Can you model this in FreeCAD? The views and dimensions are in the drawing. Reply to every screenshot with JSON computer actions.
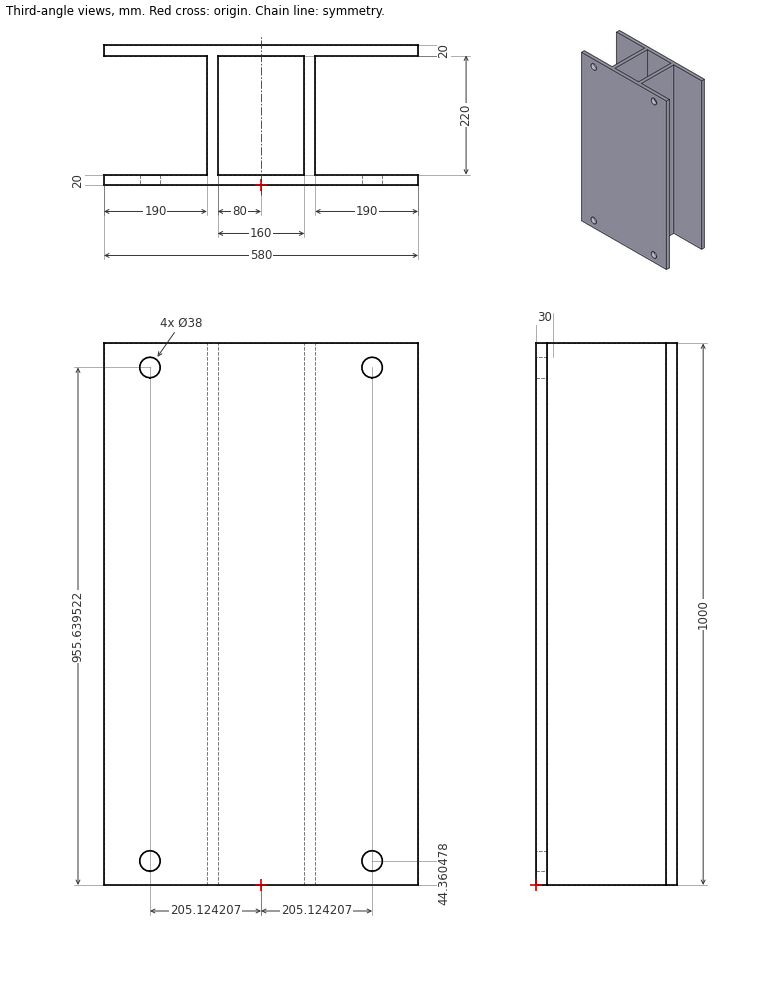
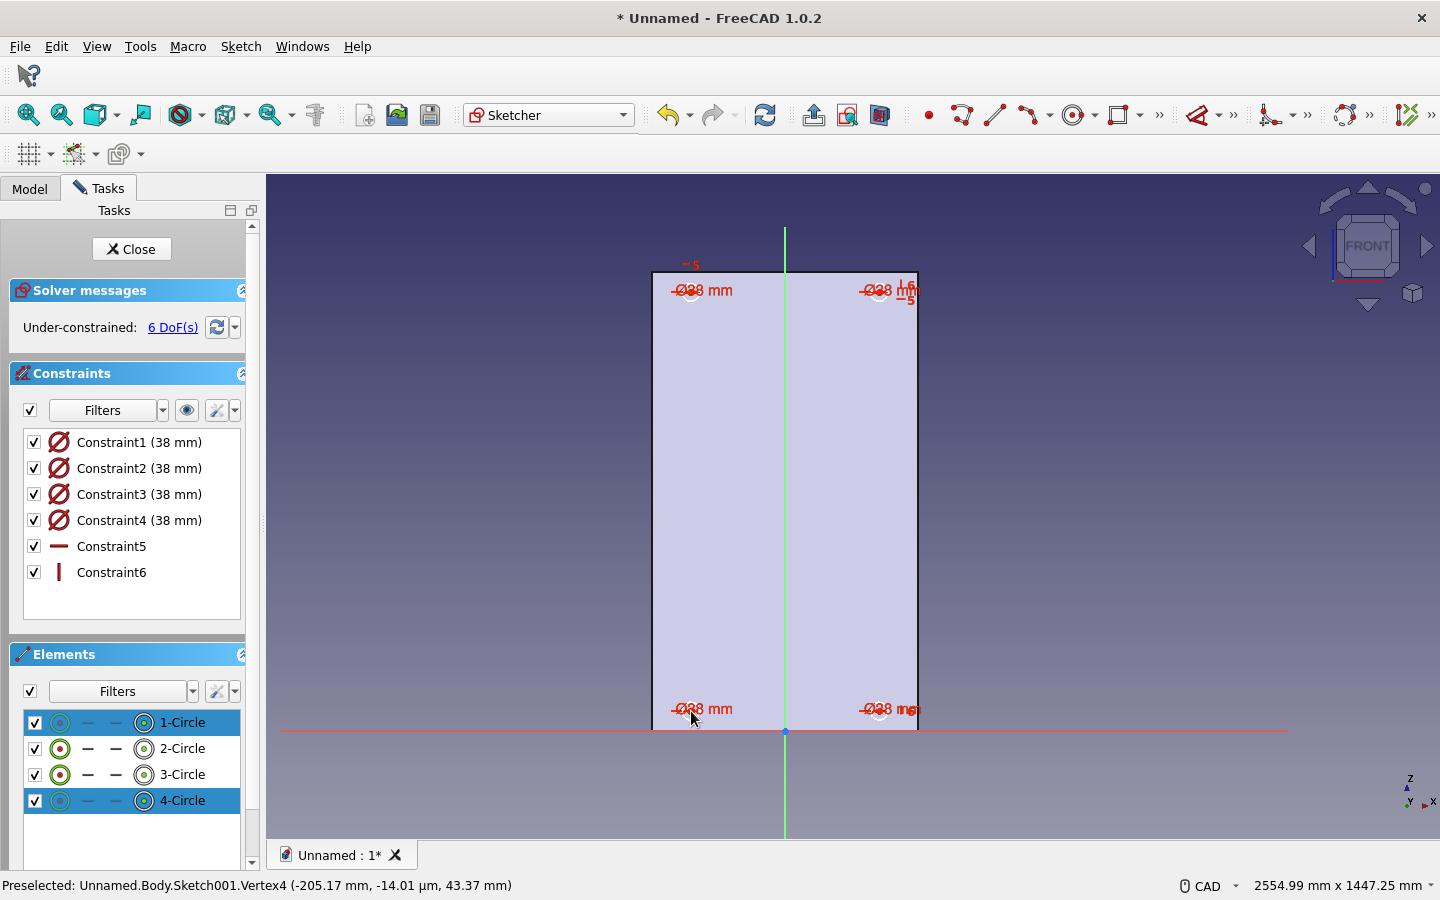
{"action": "key", "text": "v"}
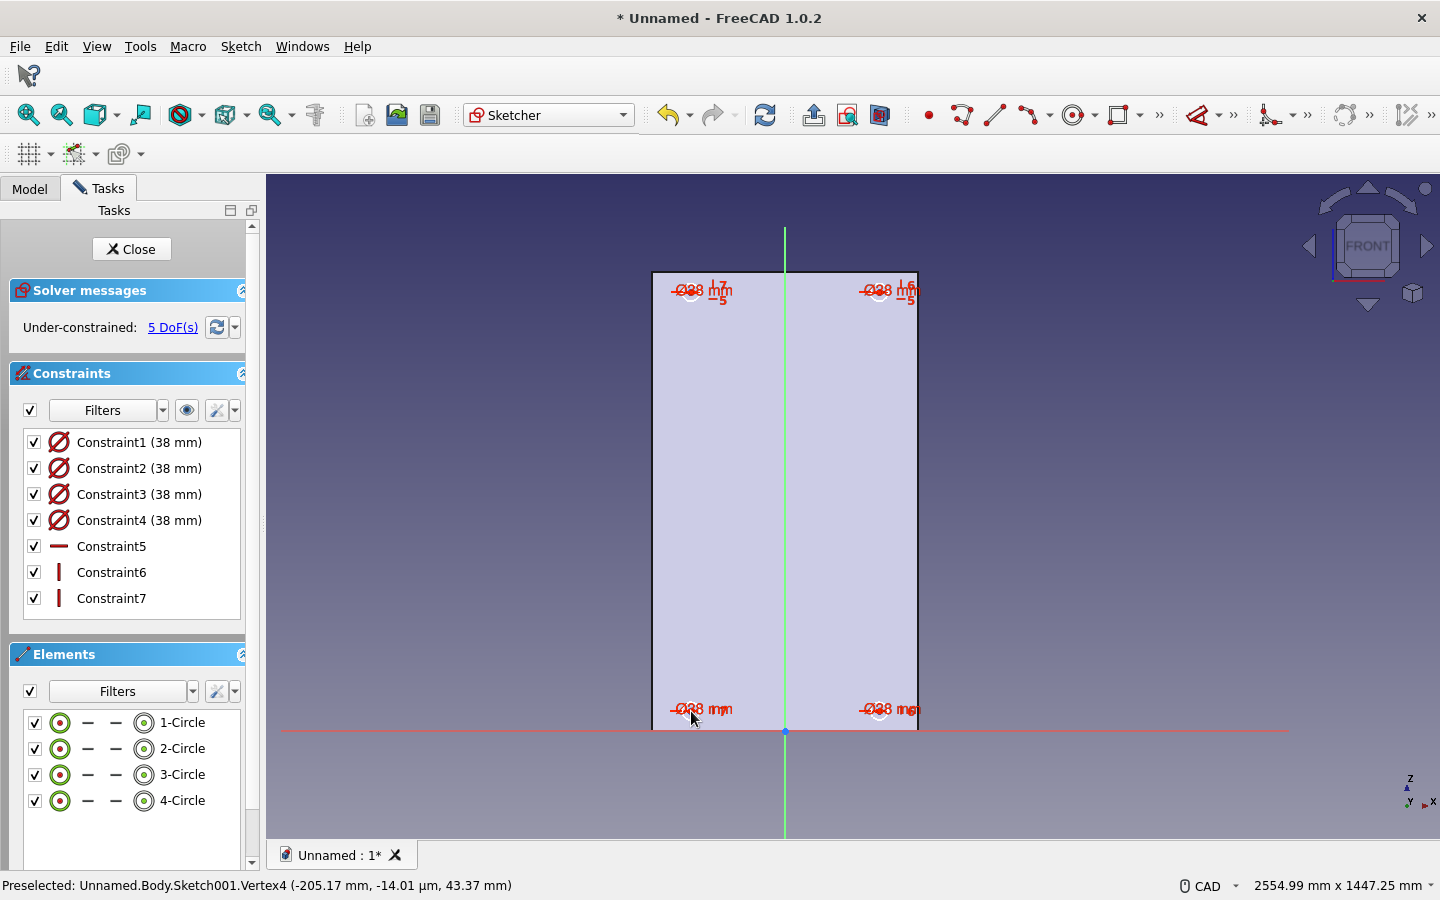
{"action": "left_click", "coordinate": [879, 711]}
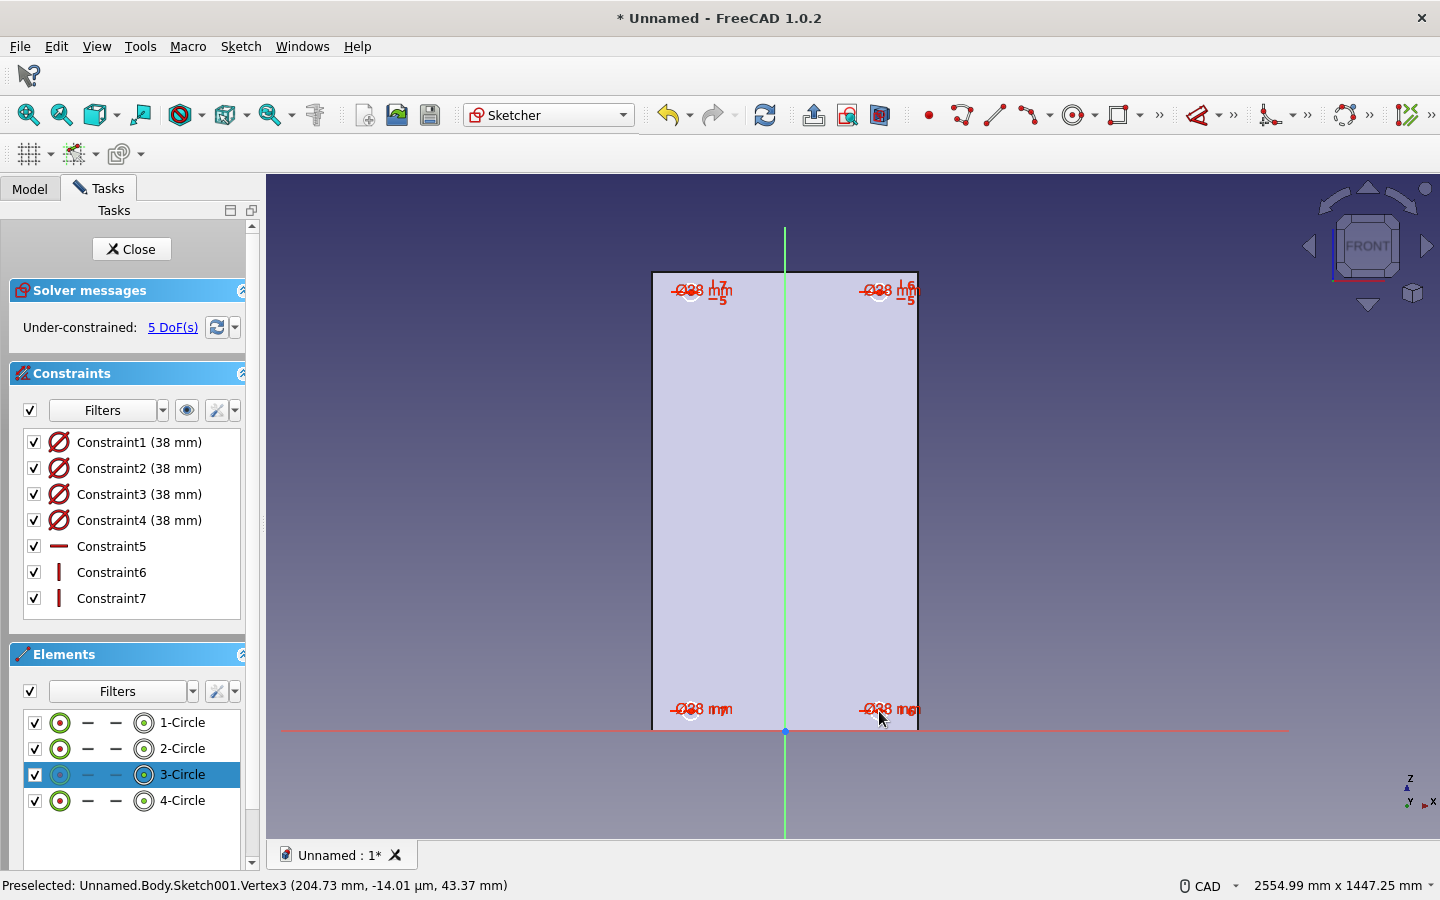
{"action": "left_click", "coordinate": [691, 711]}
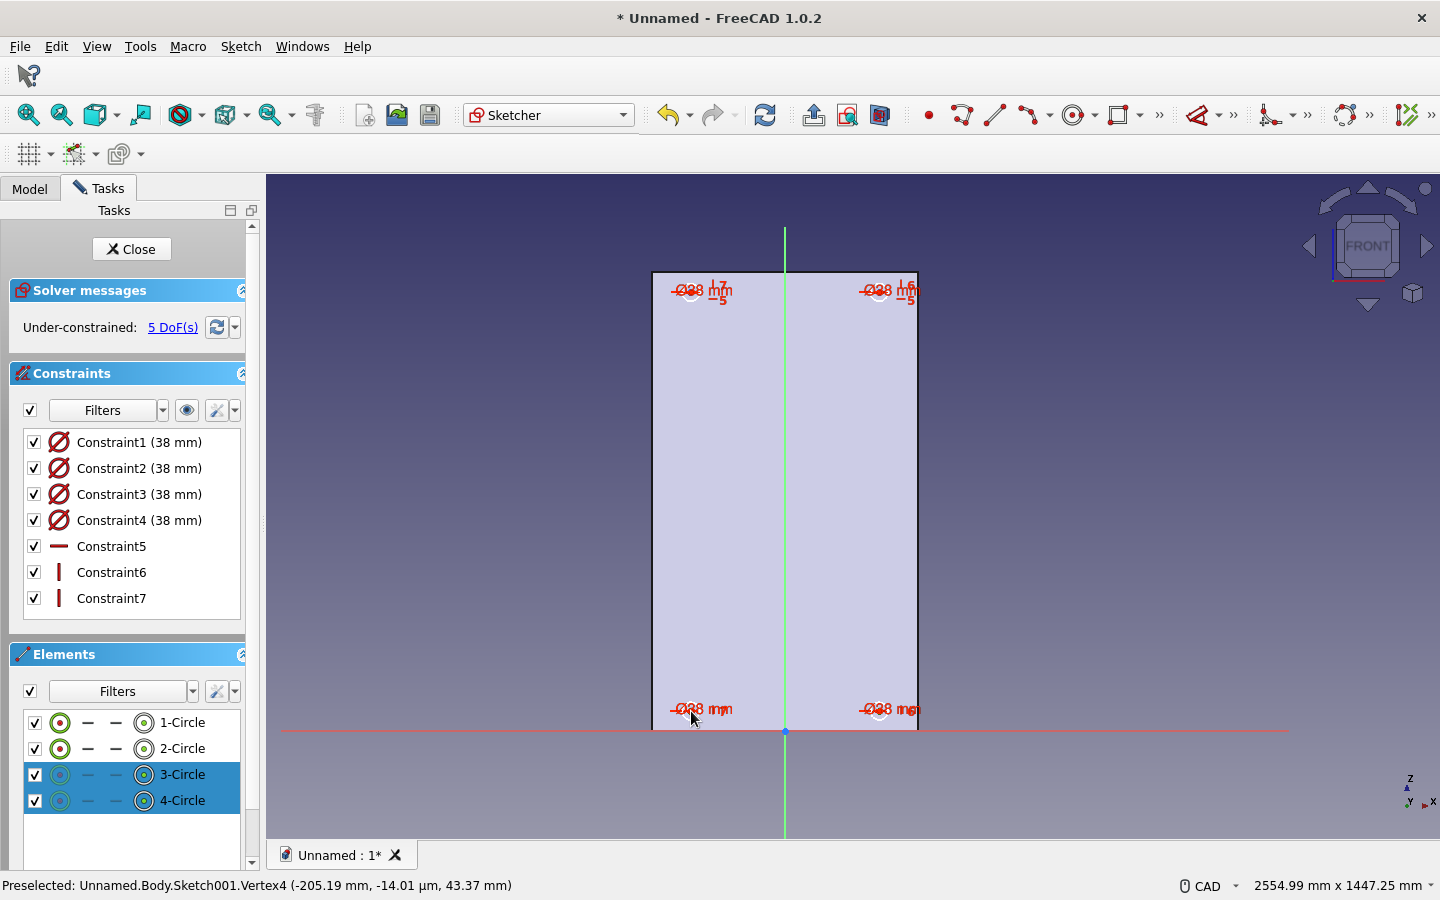
{"action": "key", "text": "h"}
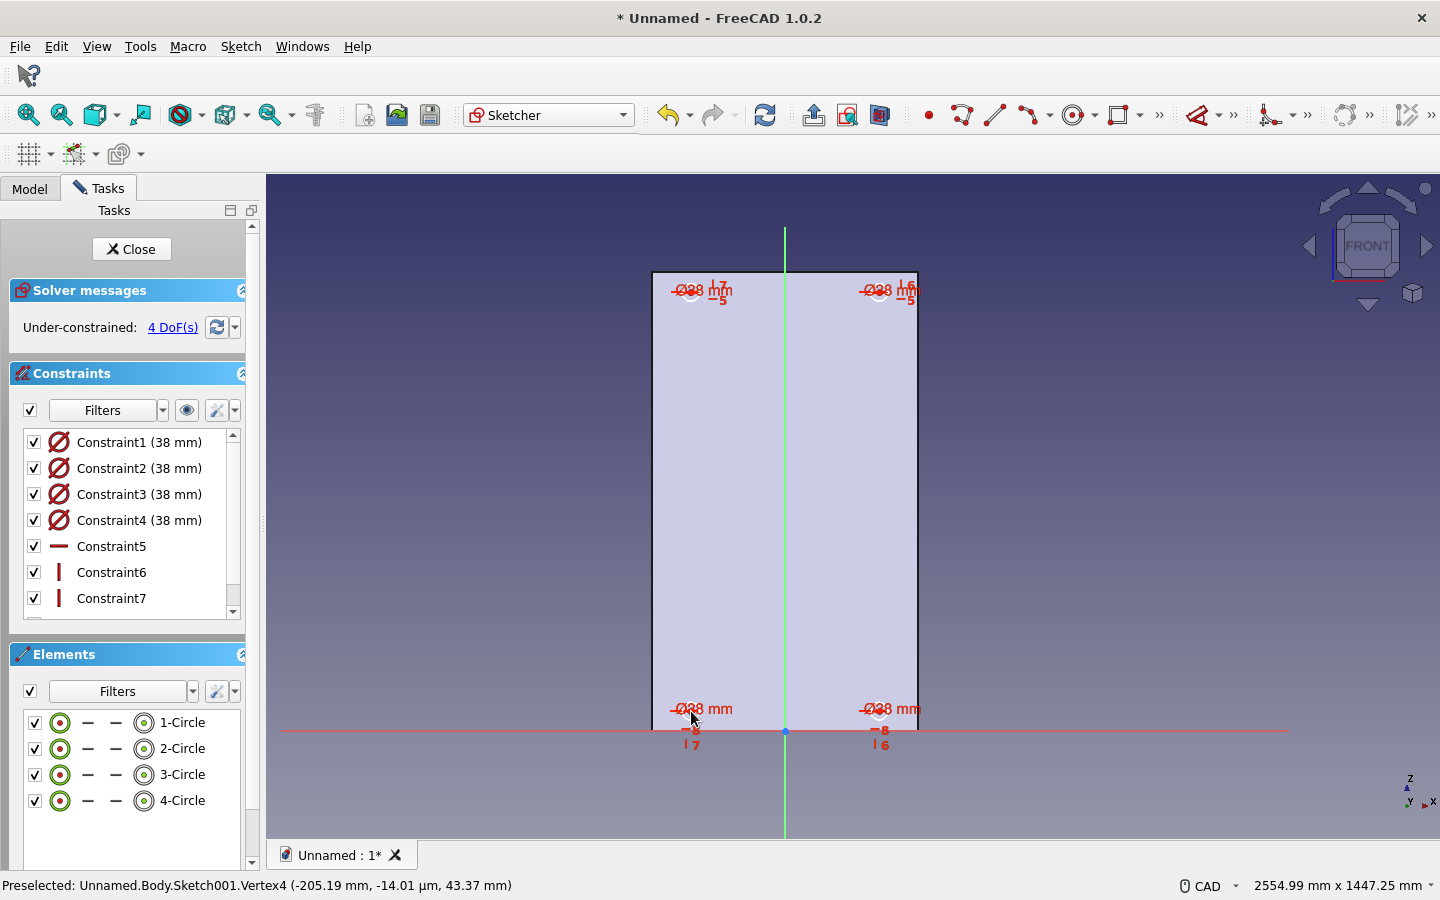
{"action": "key", "text": "d"}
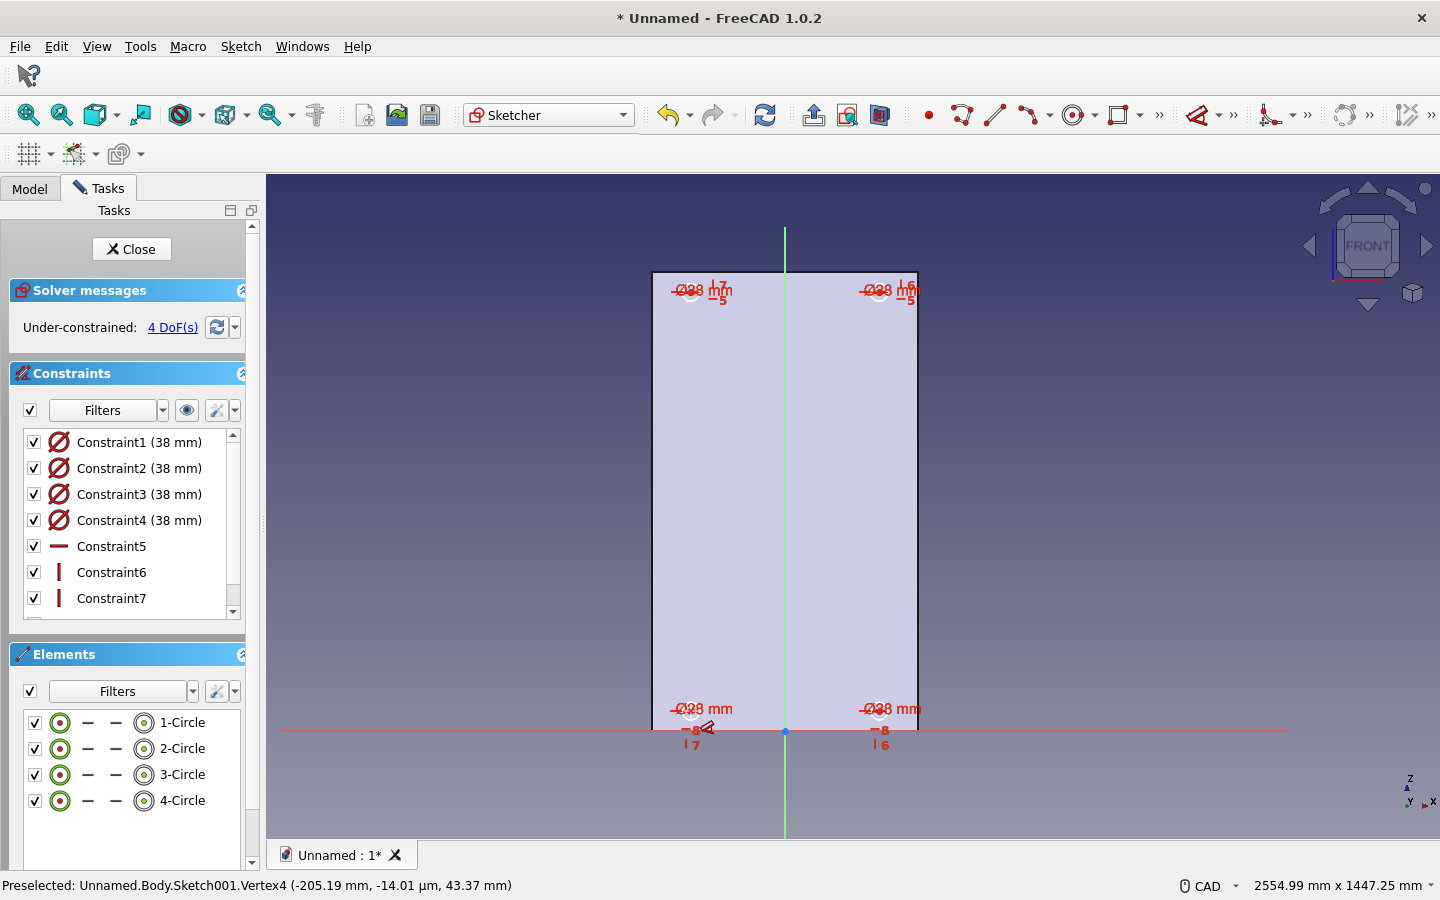
{"action": "scroll", "coordinate": [879, 711], "scroll_direction": "up", "scroll_amount": 4}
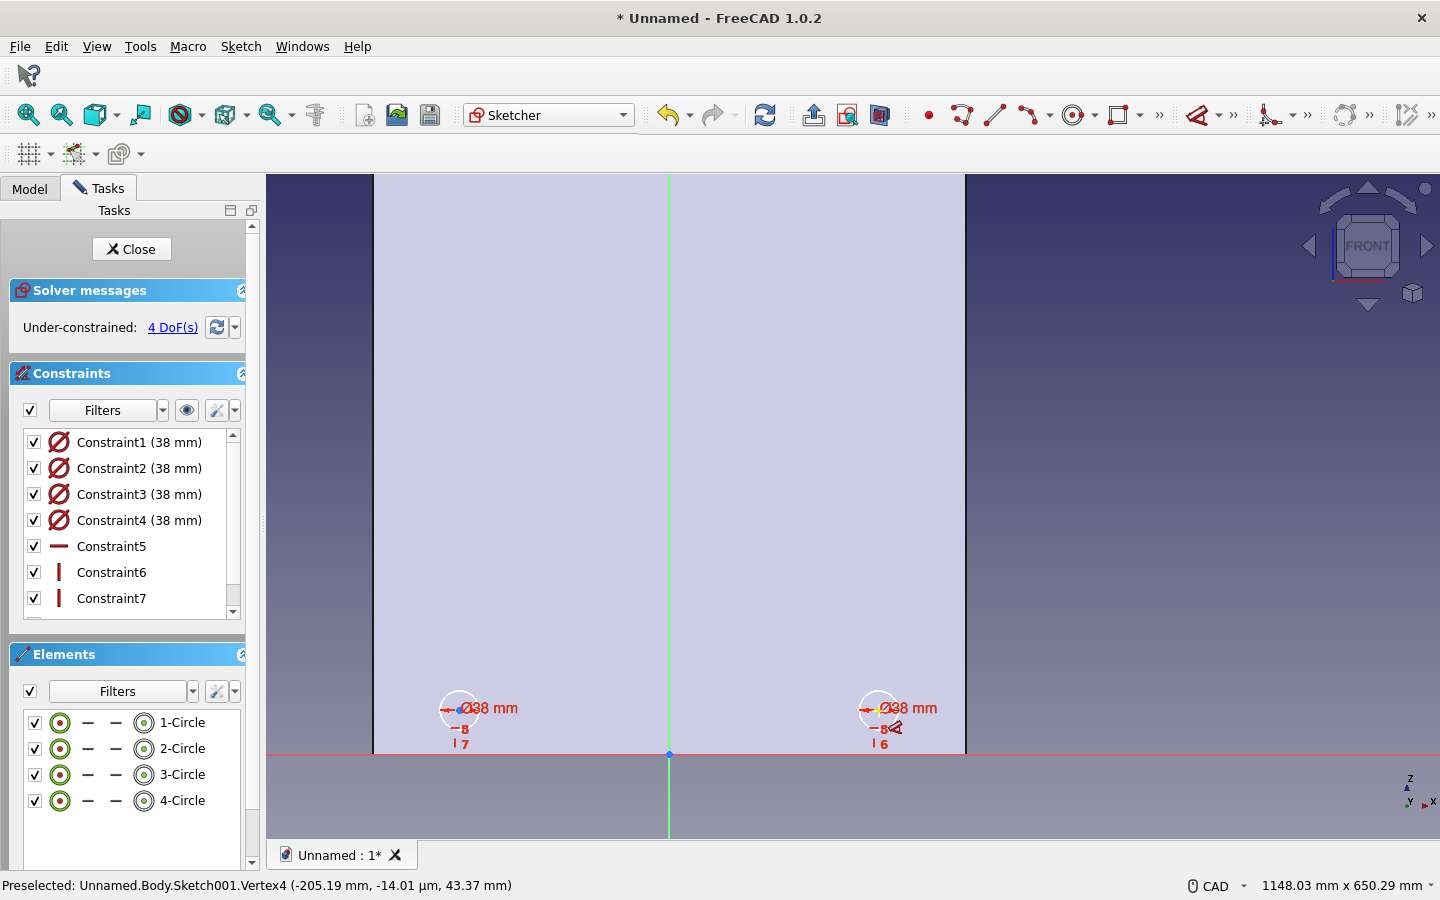
{"action": "left_click", "coordinate": [879, 710]}
{"action": "left_click", "coordinate": [913, 733]}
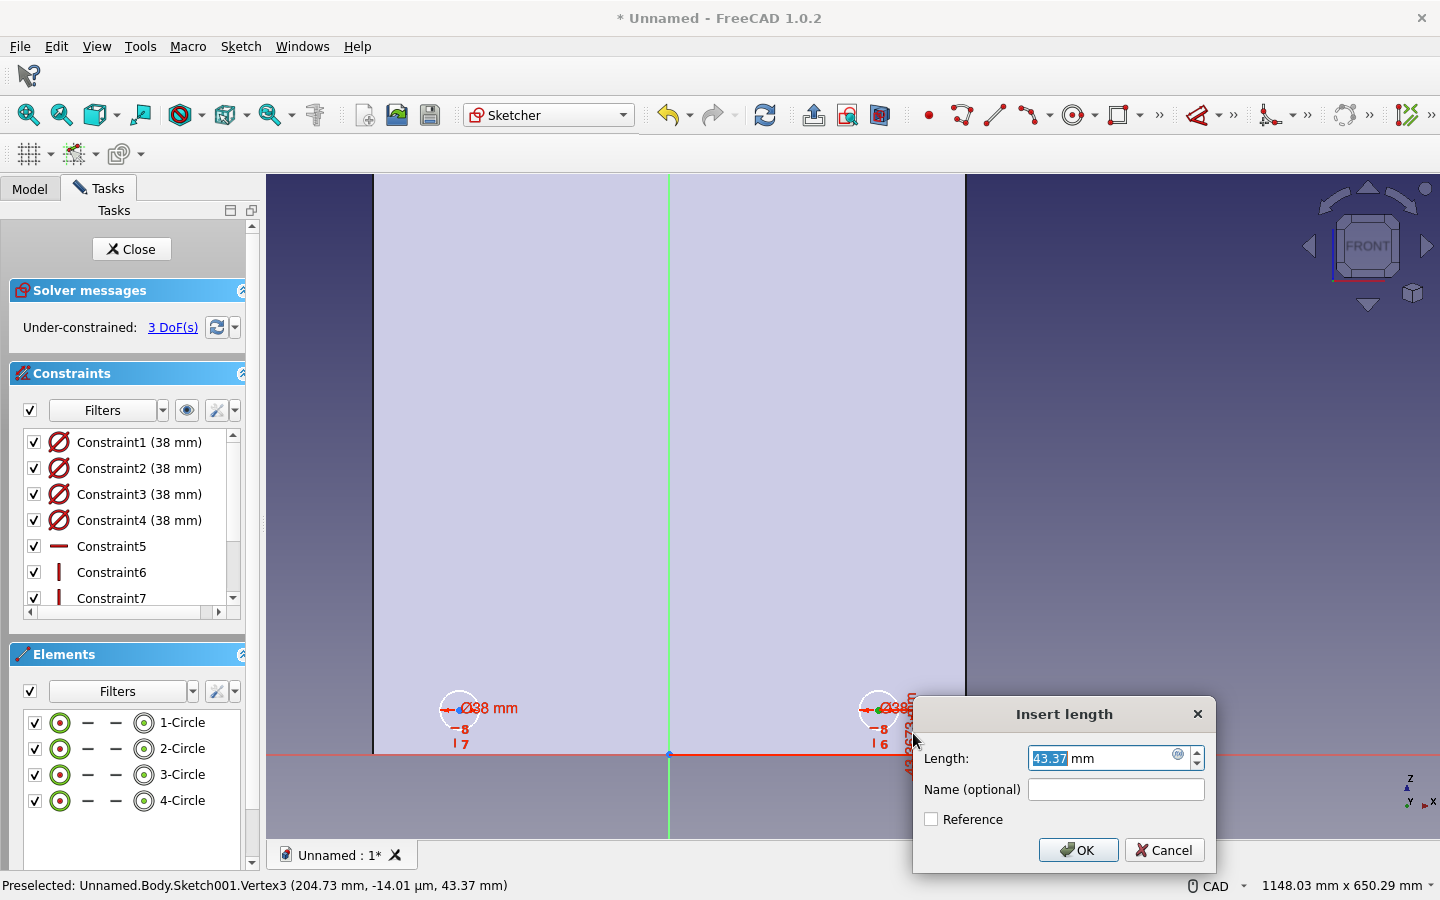
{"action": "type", "text": "44.360478"}
{"action": "key", "text": "Return"}